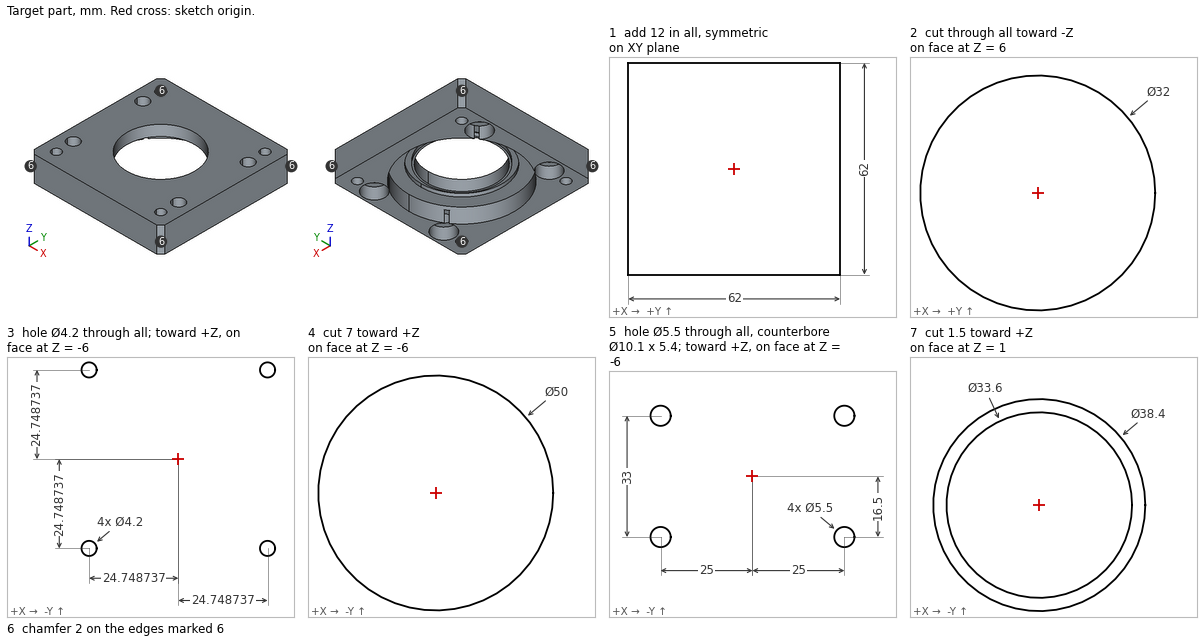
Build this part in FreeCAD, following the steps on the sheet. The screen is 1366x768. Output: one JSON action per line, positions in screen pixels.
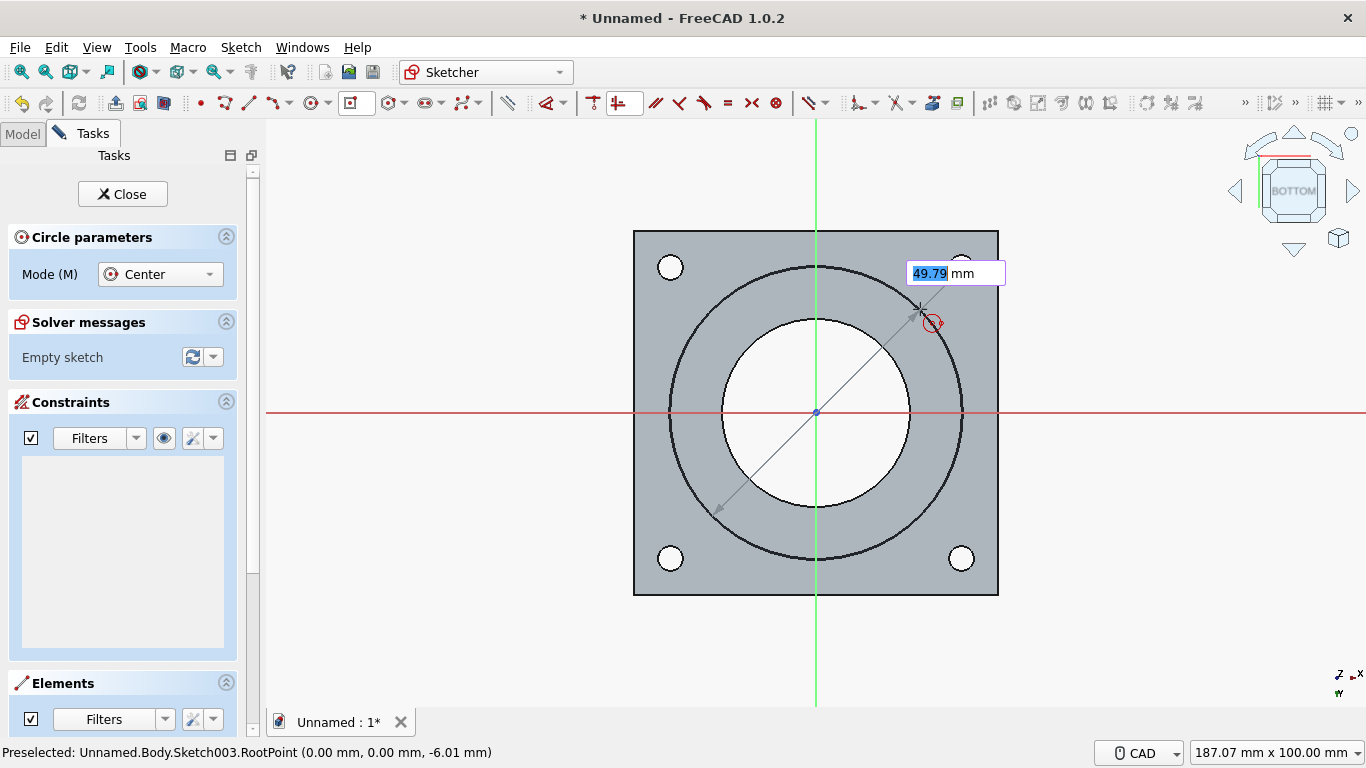
{"action": "type", "text": "50"}
{"action": "key", "text": "Return"}
{"action": "key", "text": "Escape"}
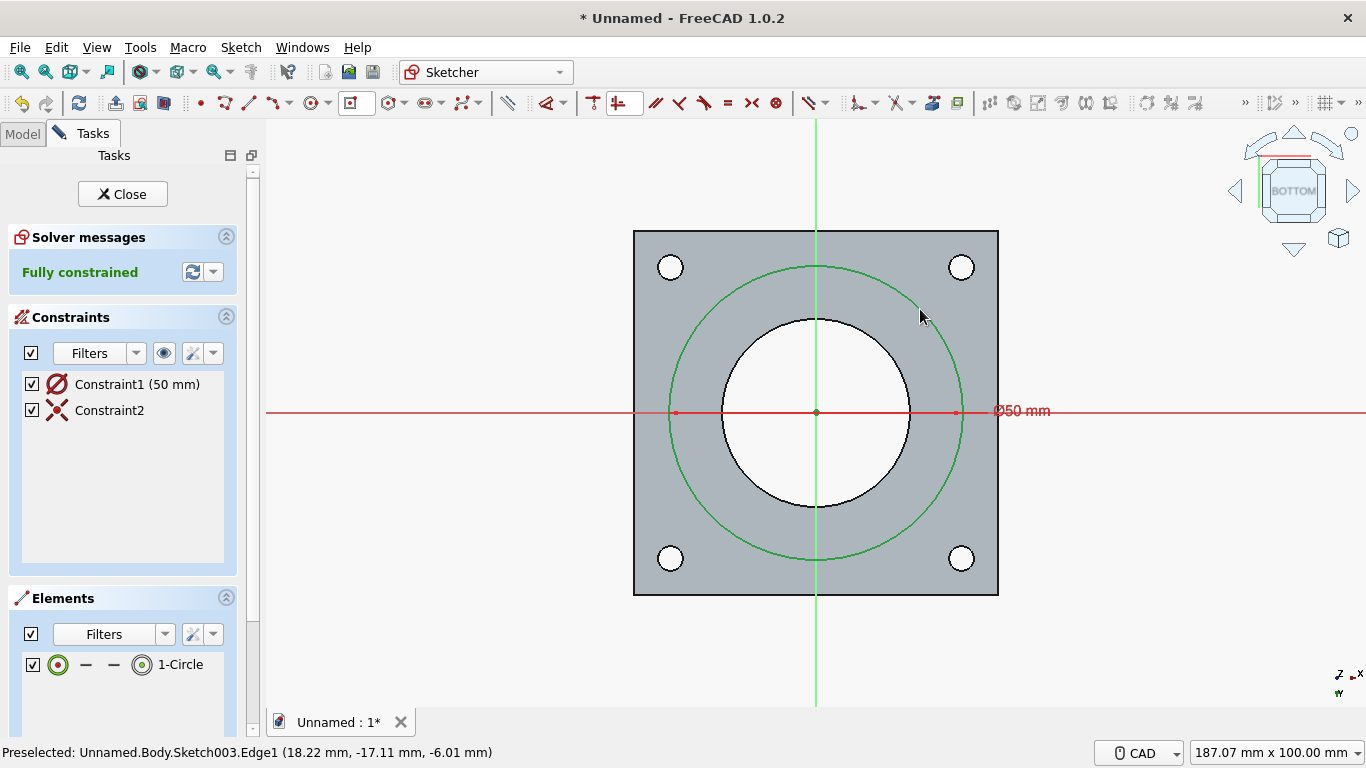
{"action": "left_click", "coordinate": [123, 194]}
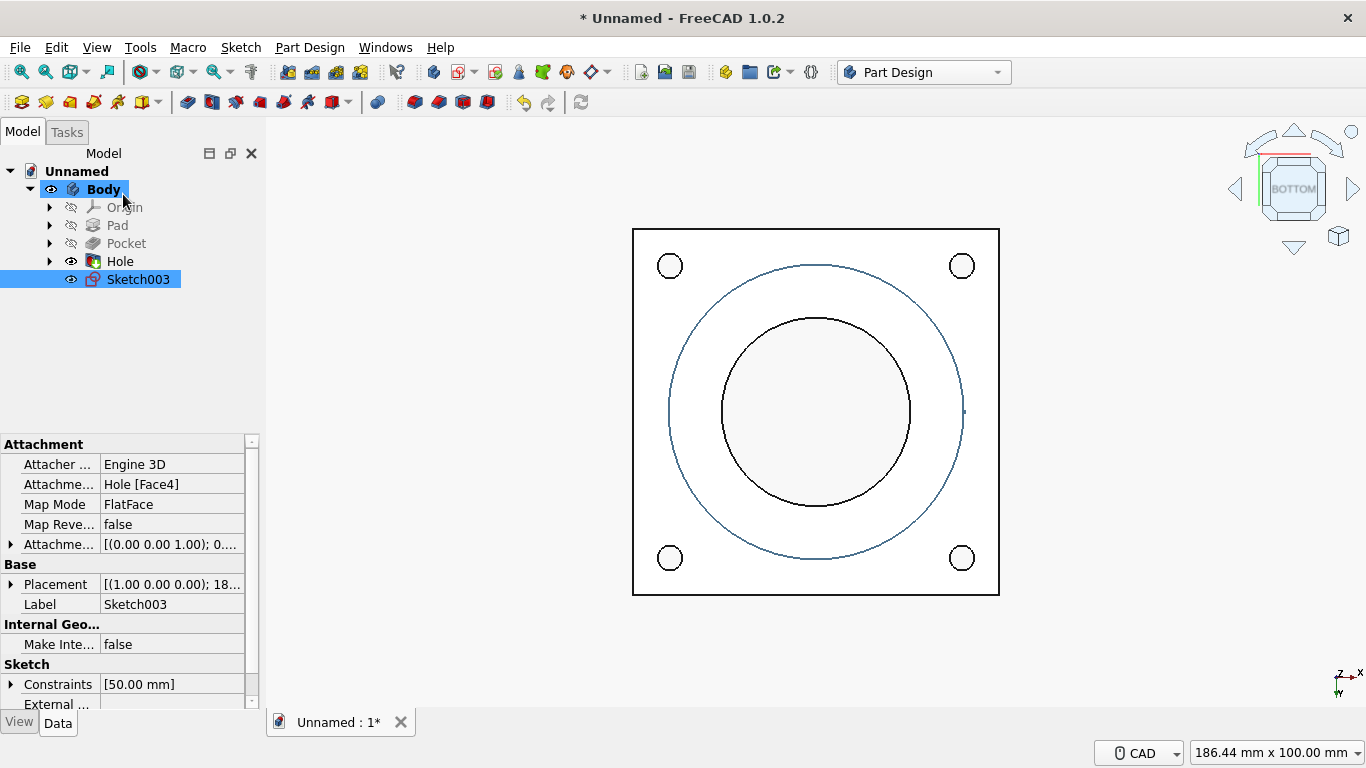
{"action": "left_click", "coordinate": [188, 102]}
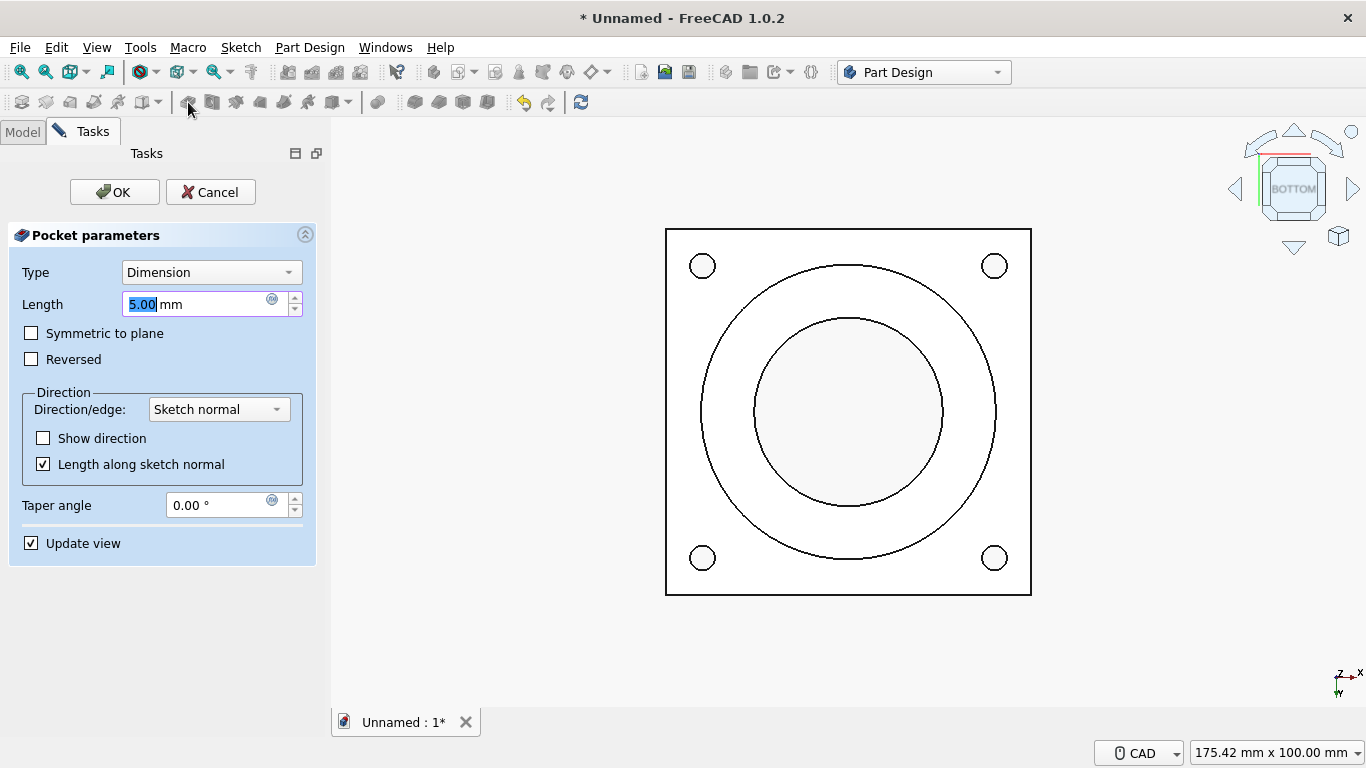
{"action": "type", "text": "7"}
{"action": "key", "text": "Tab"}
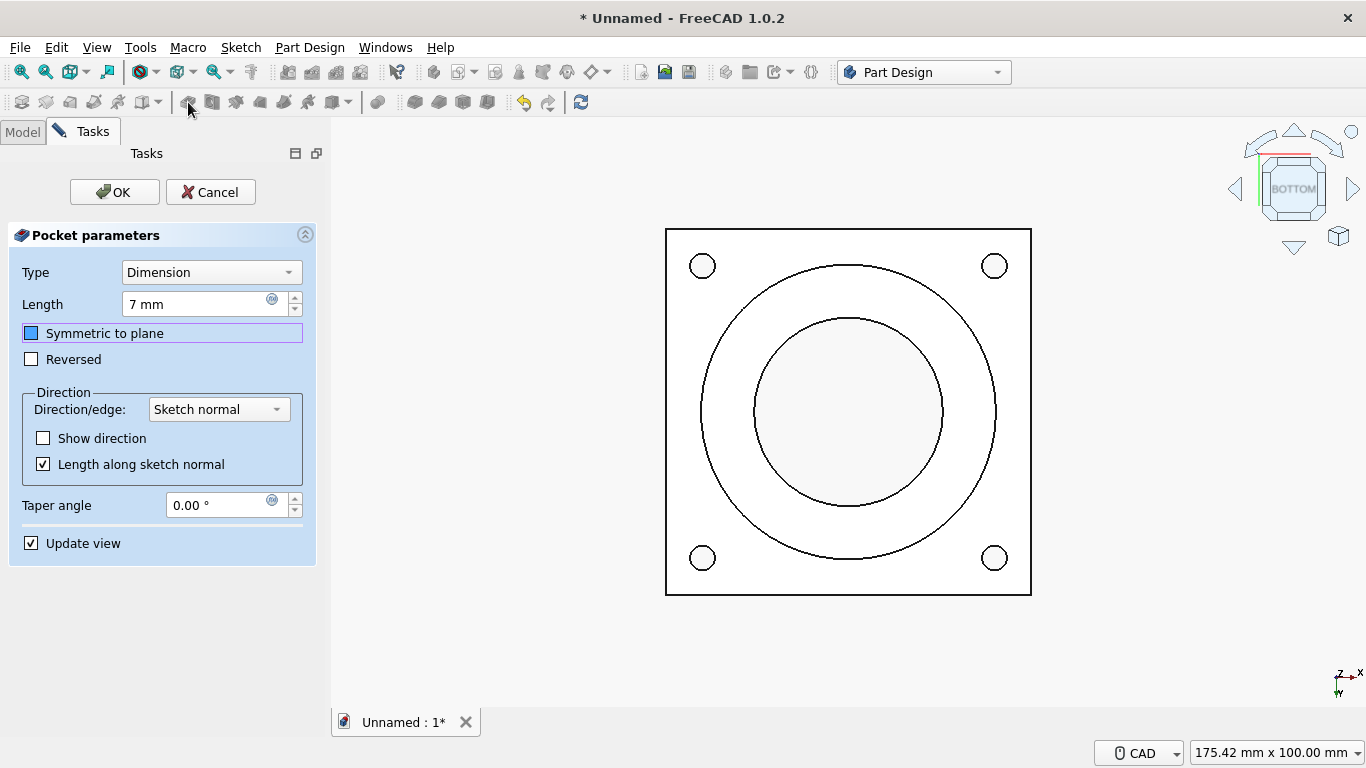
{"action": "left_click", "coordinate": [115, 192]}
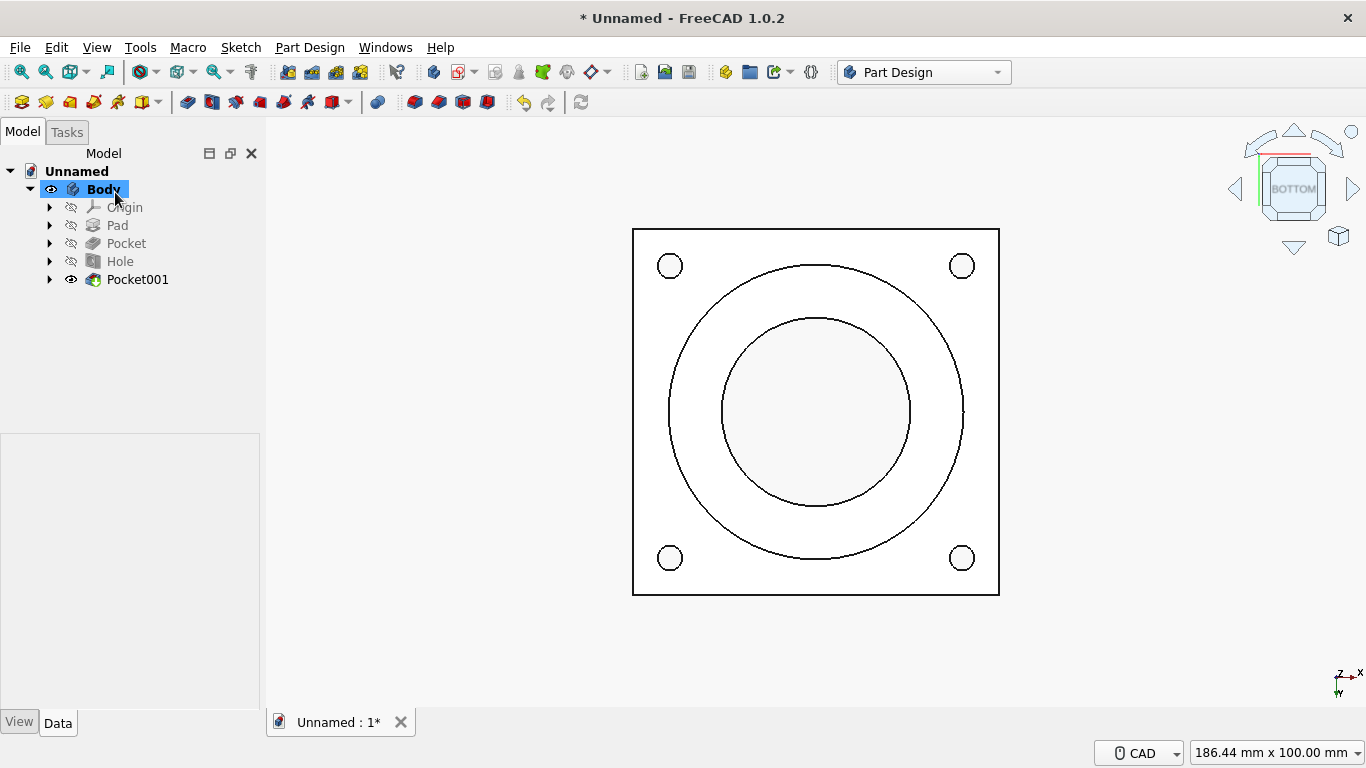
{"action": "left_click", "coordinate": [973, 516]}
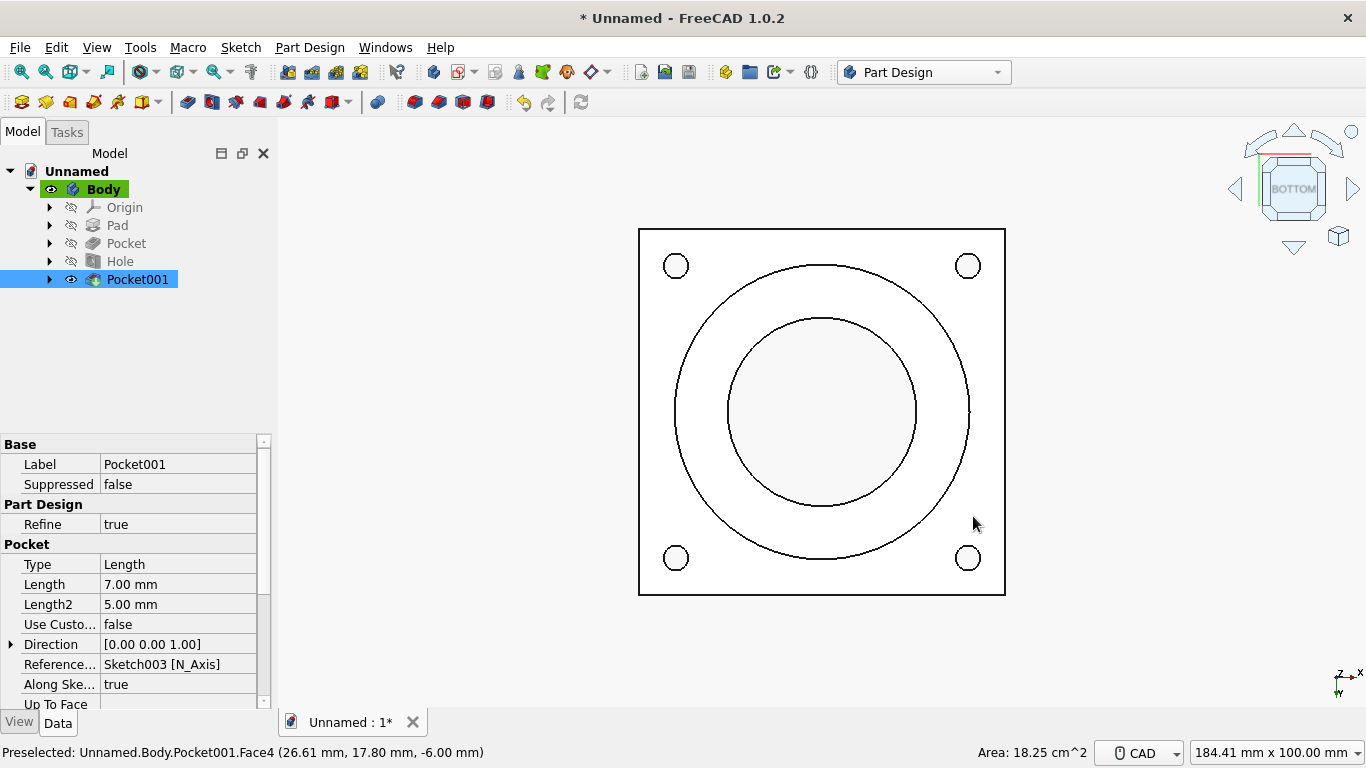
{"action": "left_click", "coordinate": [458, 72]}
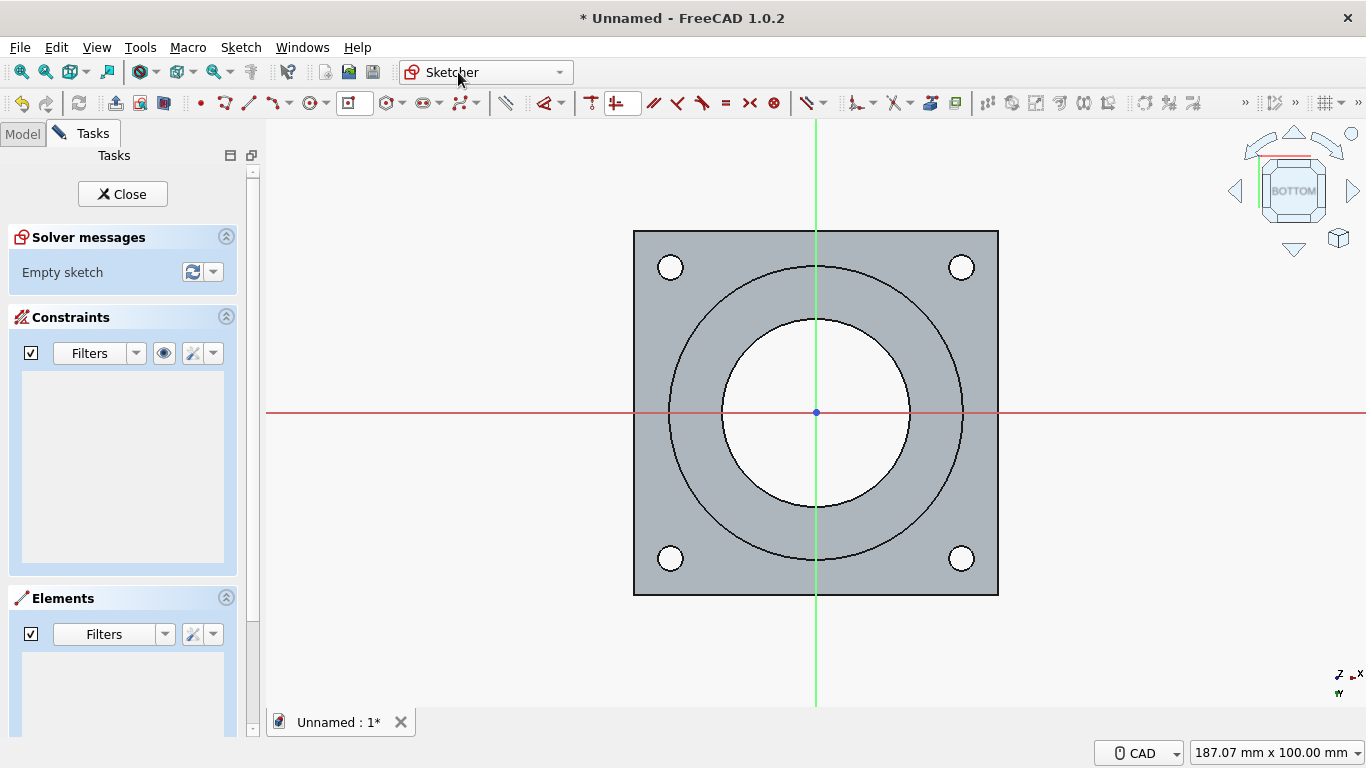
{"action": "scroll", "coordinate": [899, 413], "scroll_direction": "up", "scroll_amount": 3}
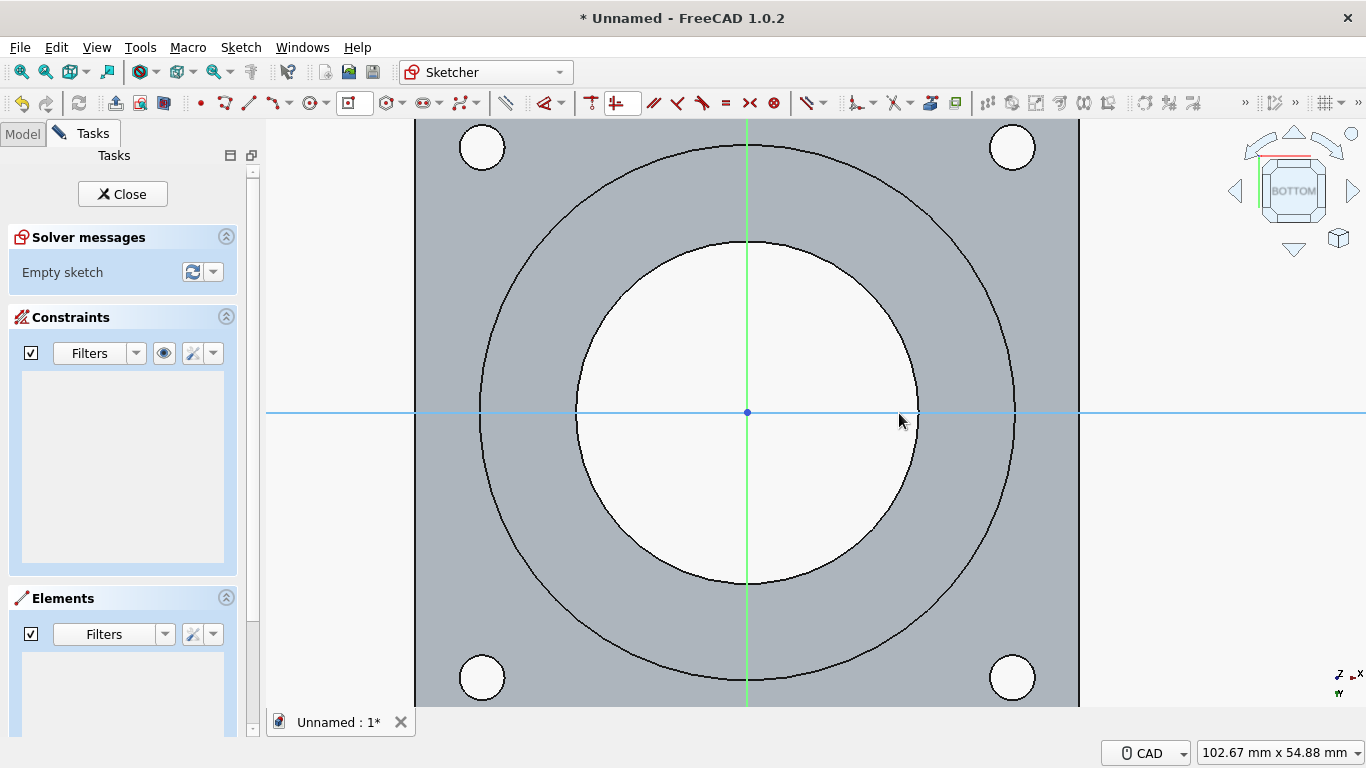
{"action": "left_click", "coordinate": [310, 104]}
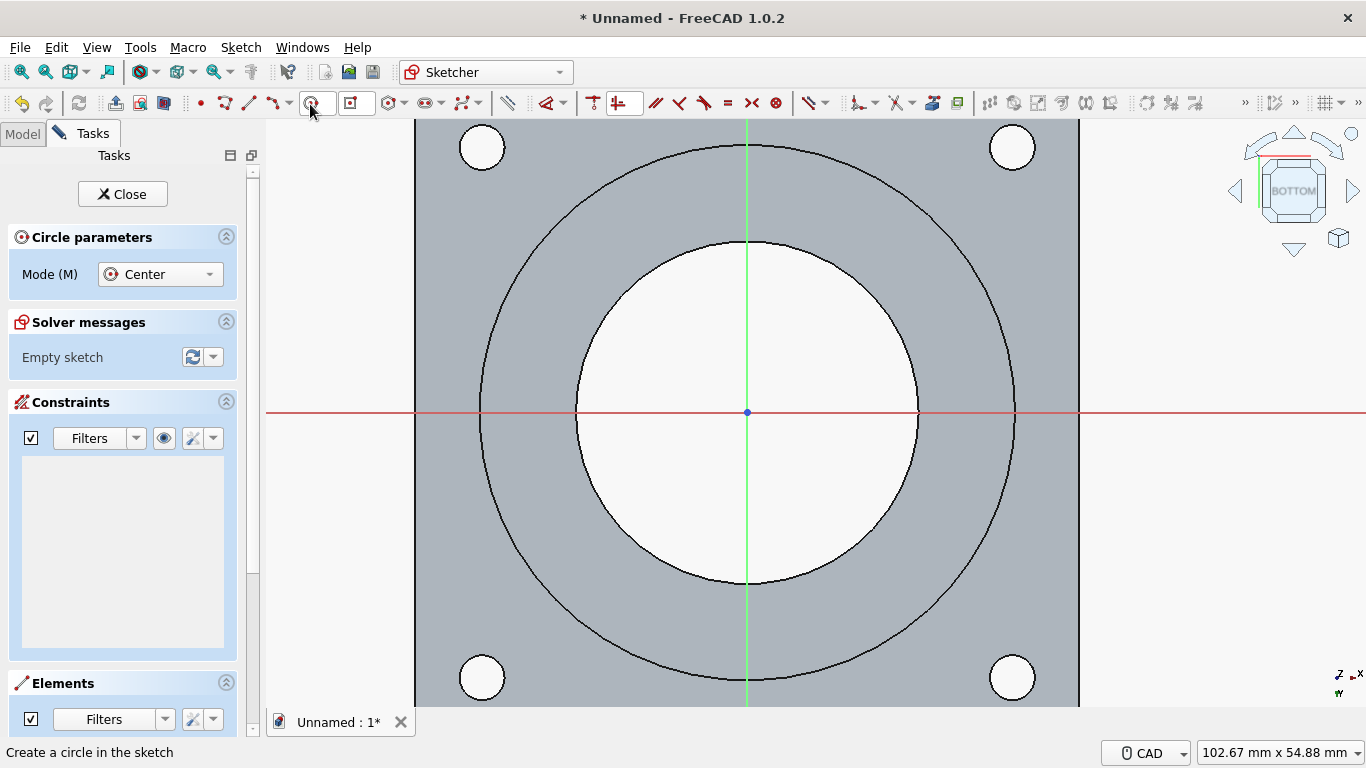
{"action": "left_click", "coordinate": [1015, 589]}
{"action": "mouse_move", "coordinate": [1036, 569]}